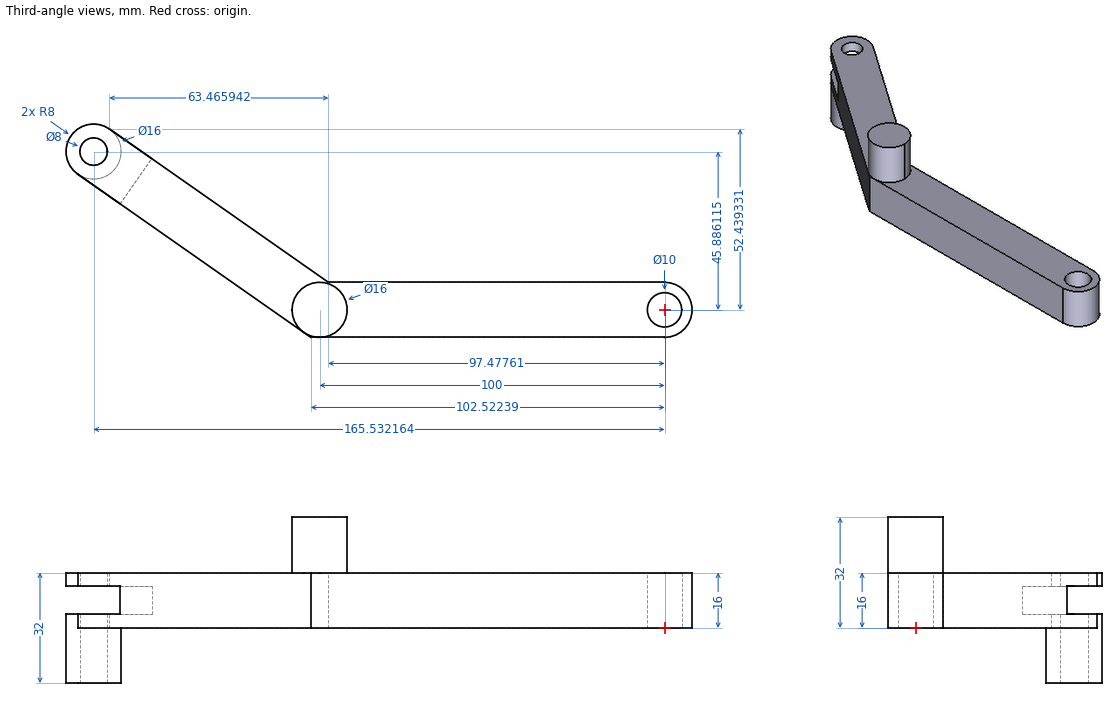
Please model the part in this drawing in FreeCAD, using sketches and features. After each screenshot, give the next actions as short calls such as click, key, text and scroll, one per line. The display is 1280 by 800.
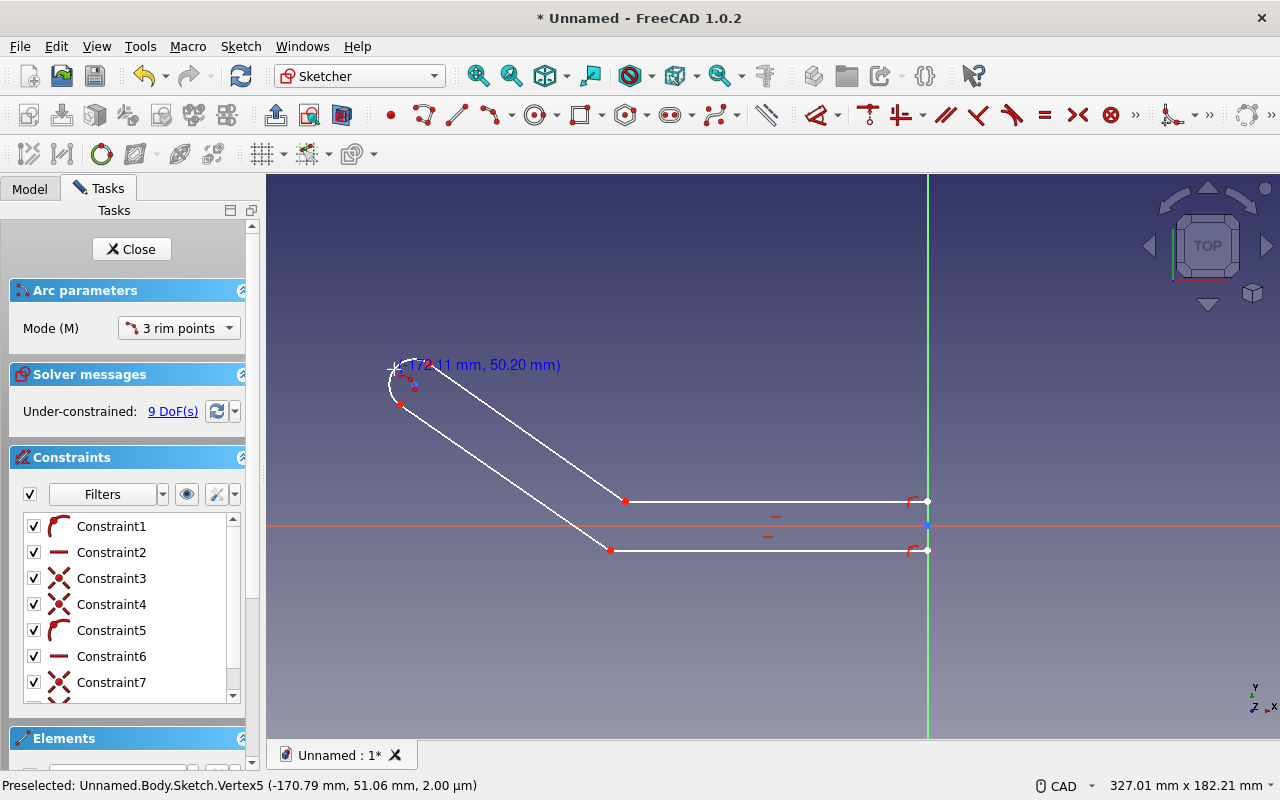
click(928, 551)
click(928, 502)
click(948, 540)
key(Escape)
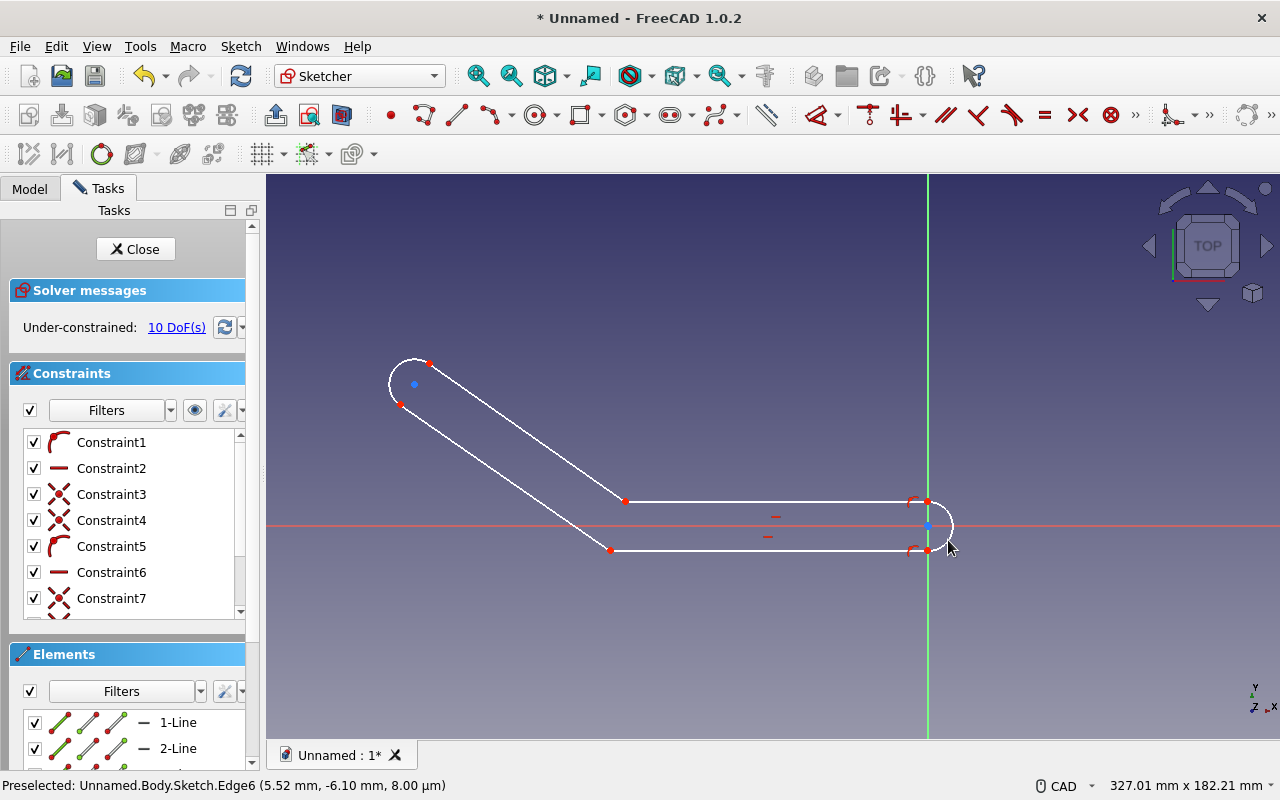
click(837, 502)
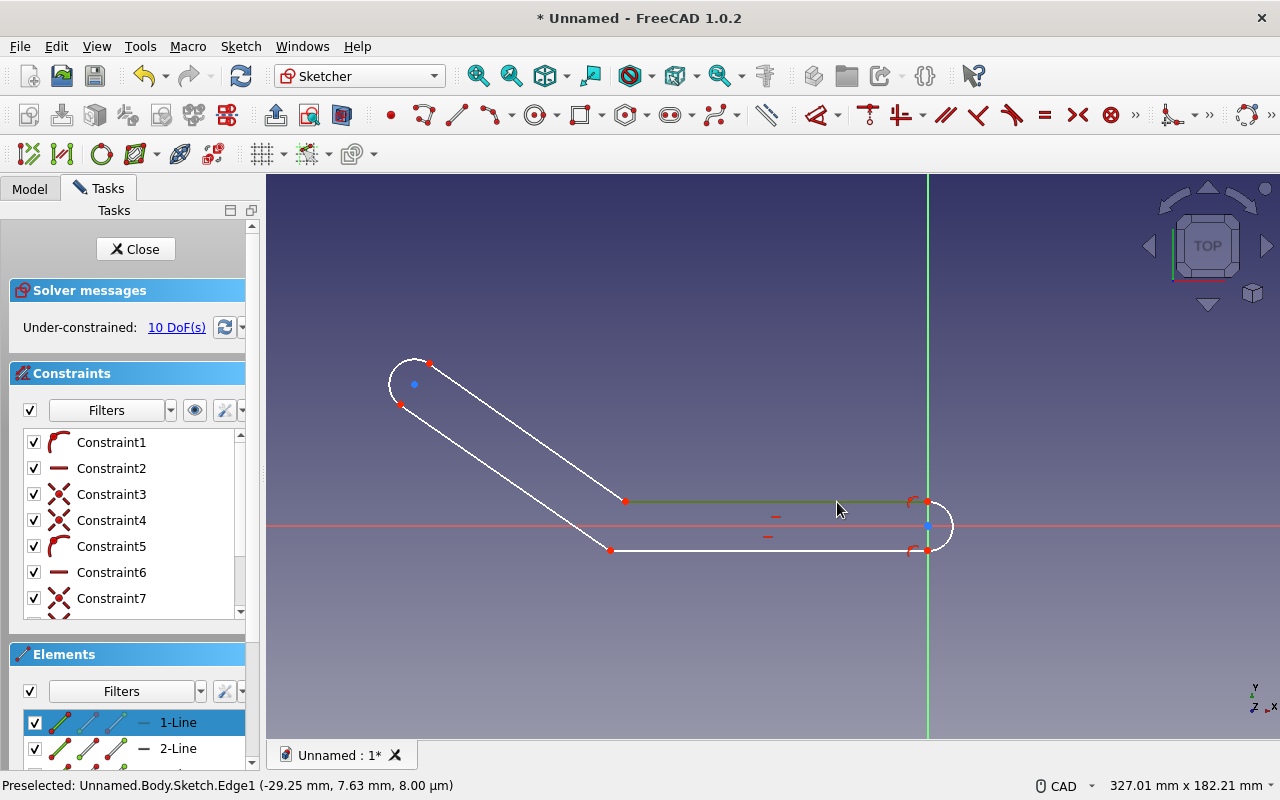
click(948, 541)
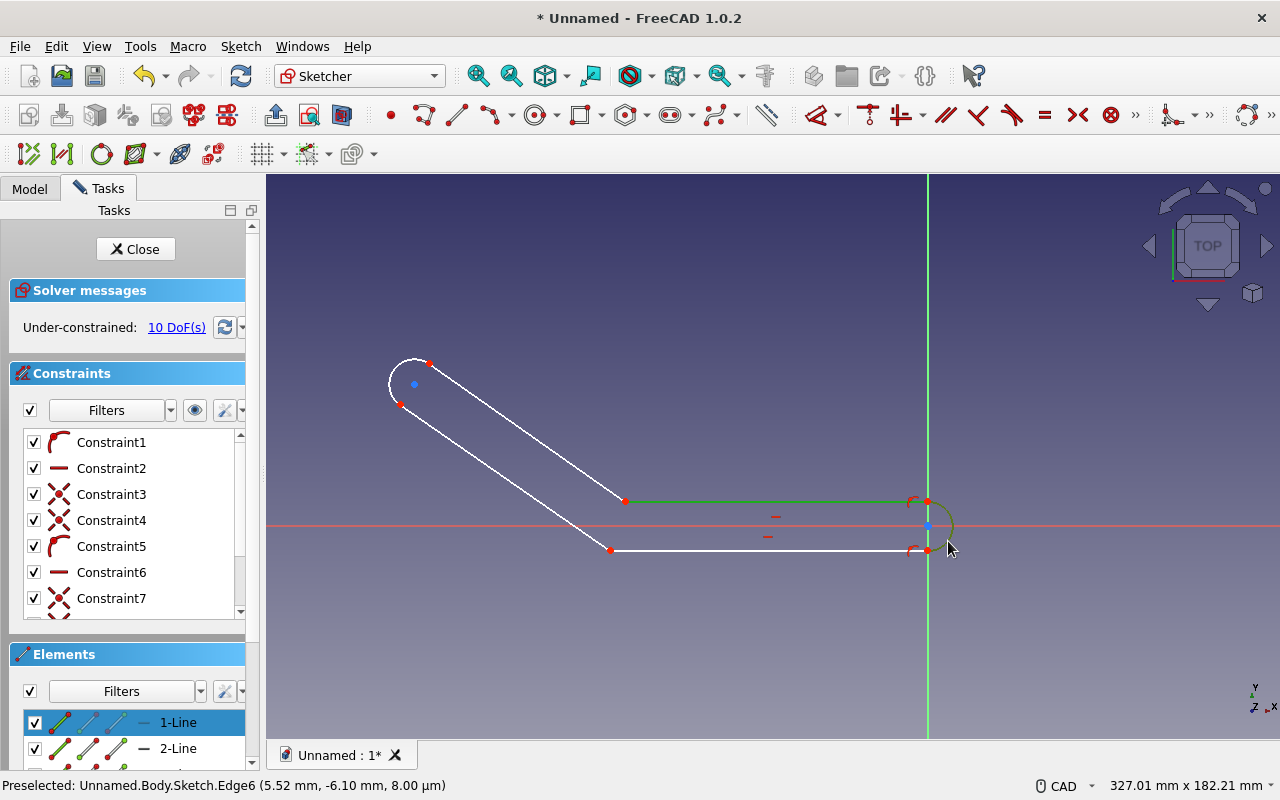
click(1012, 116)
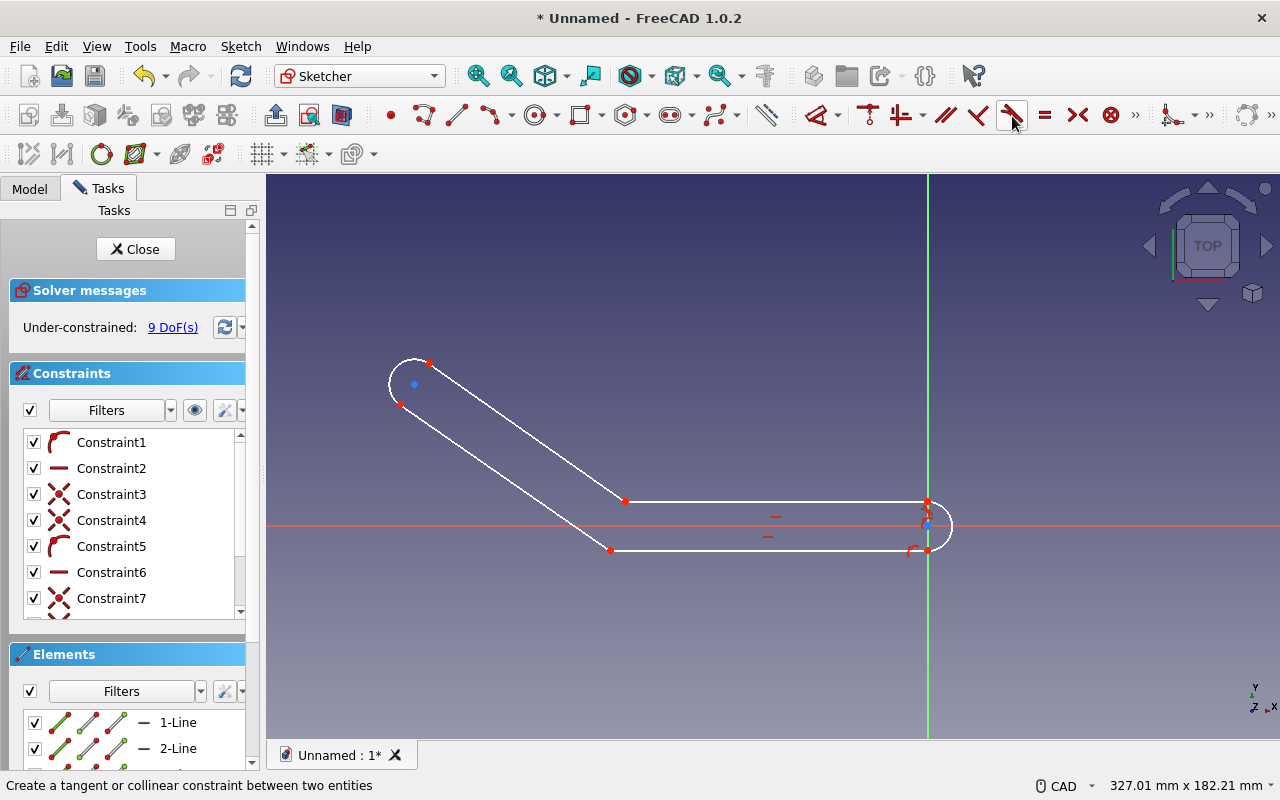
click(566, 461)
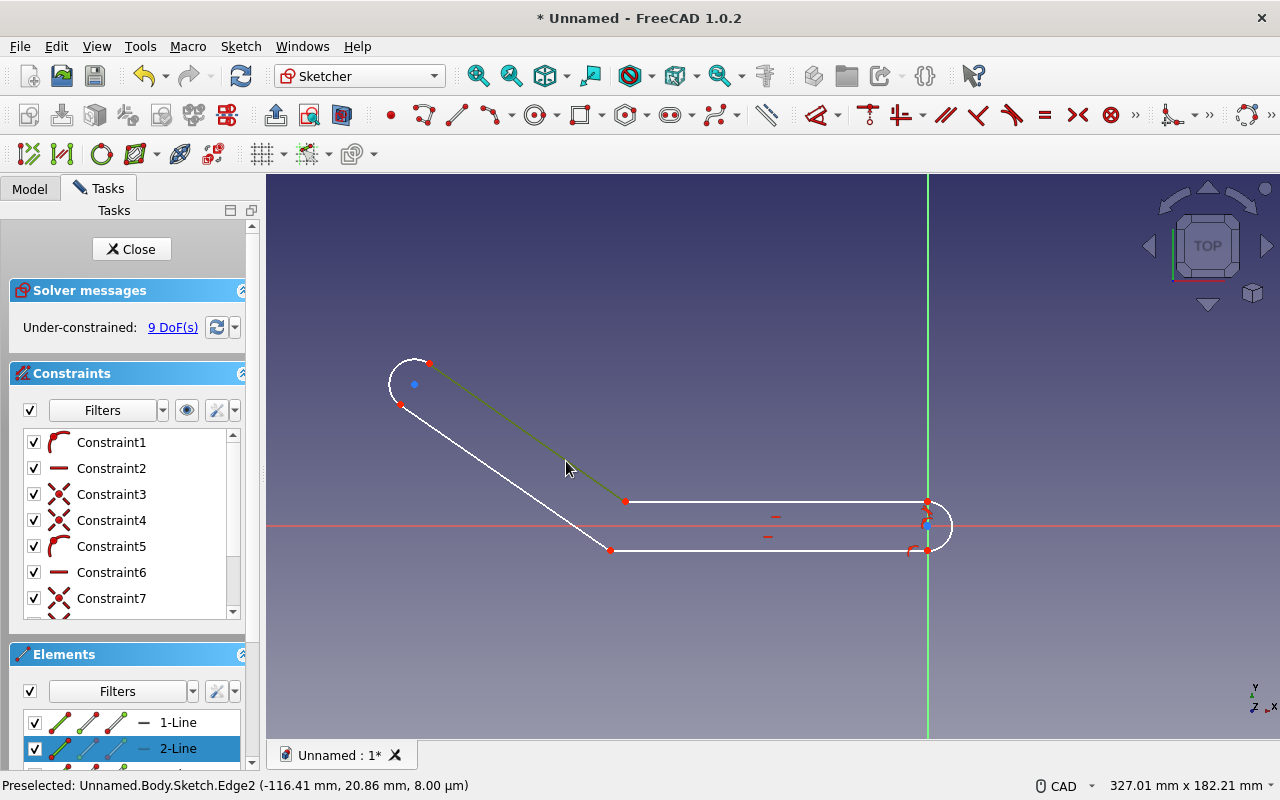
click(406, 361)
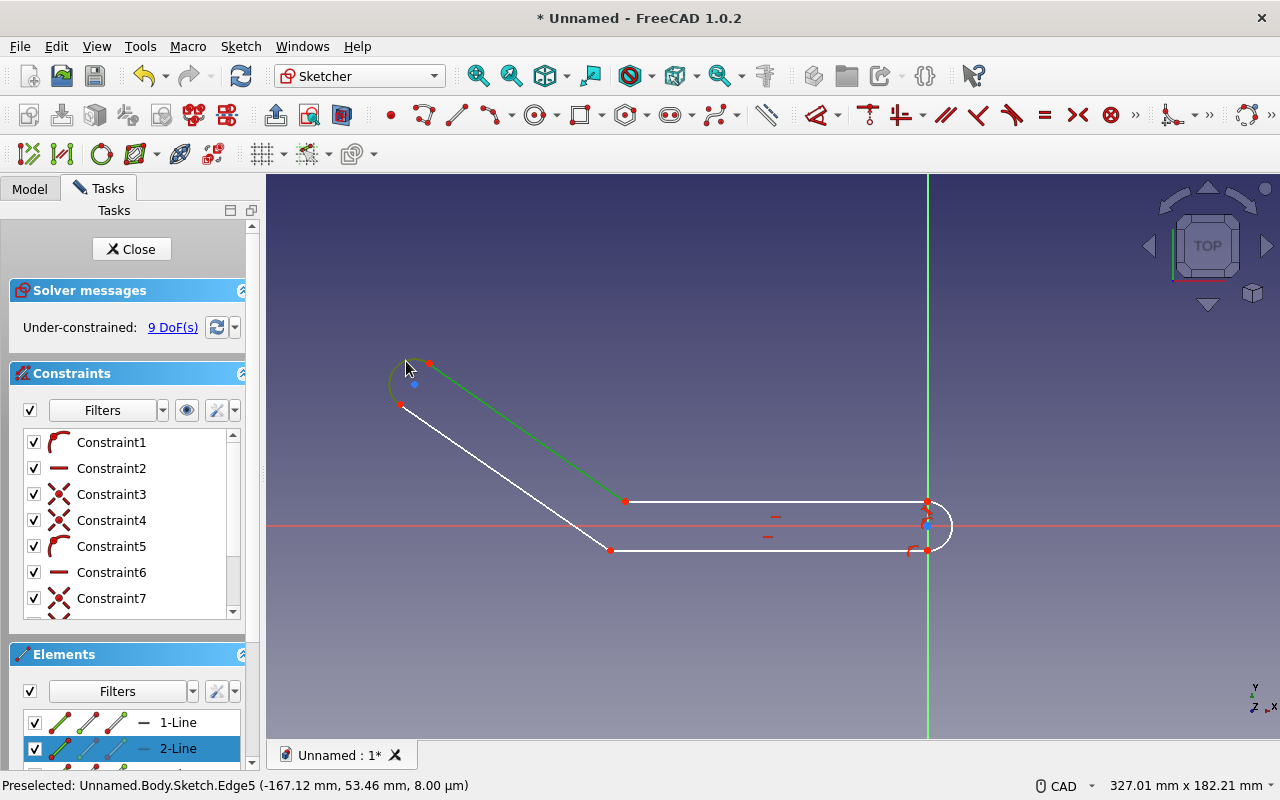
click(1012, 116)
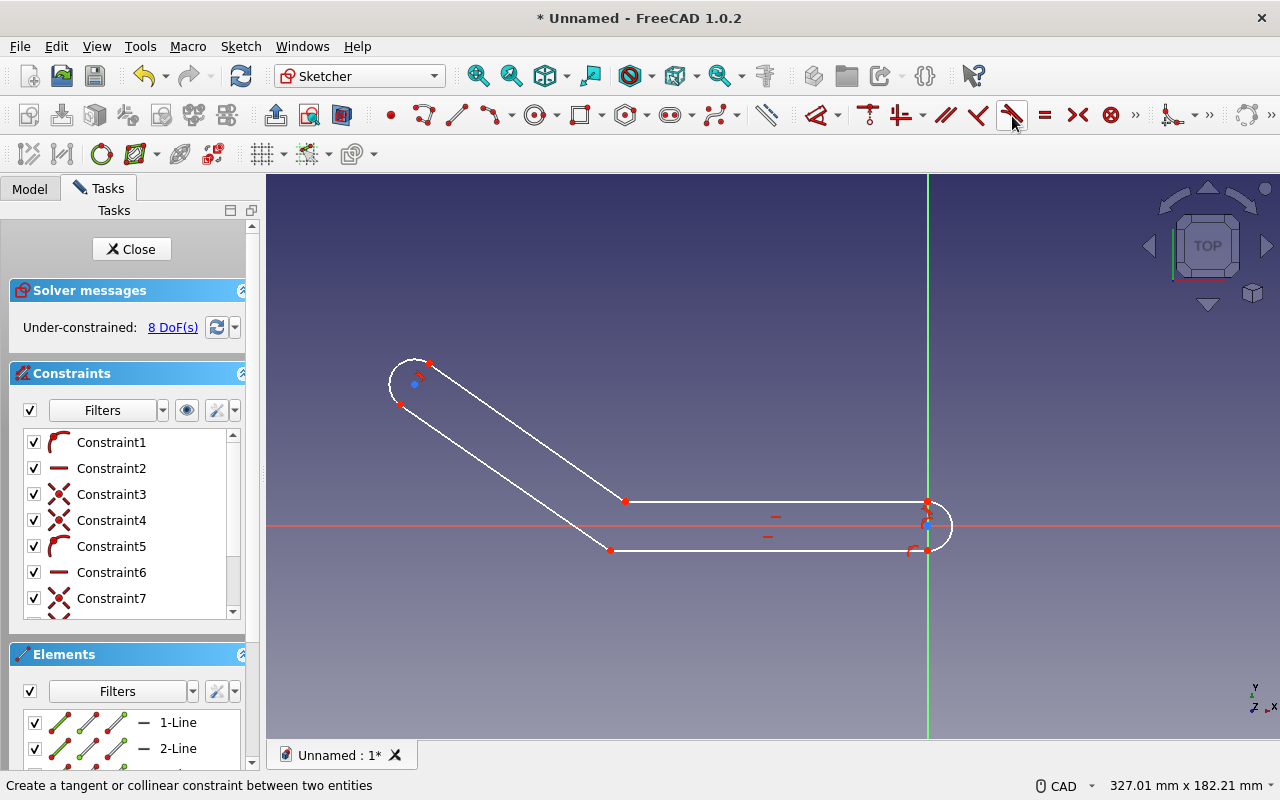
click(463, 449)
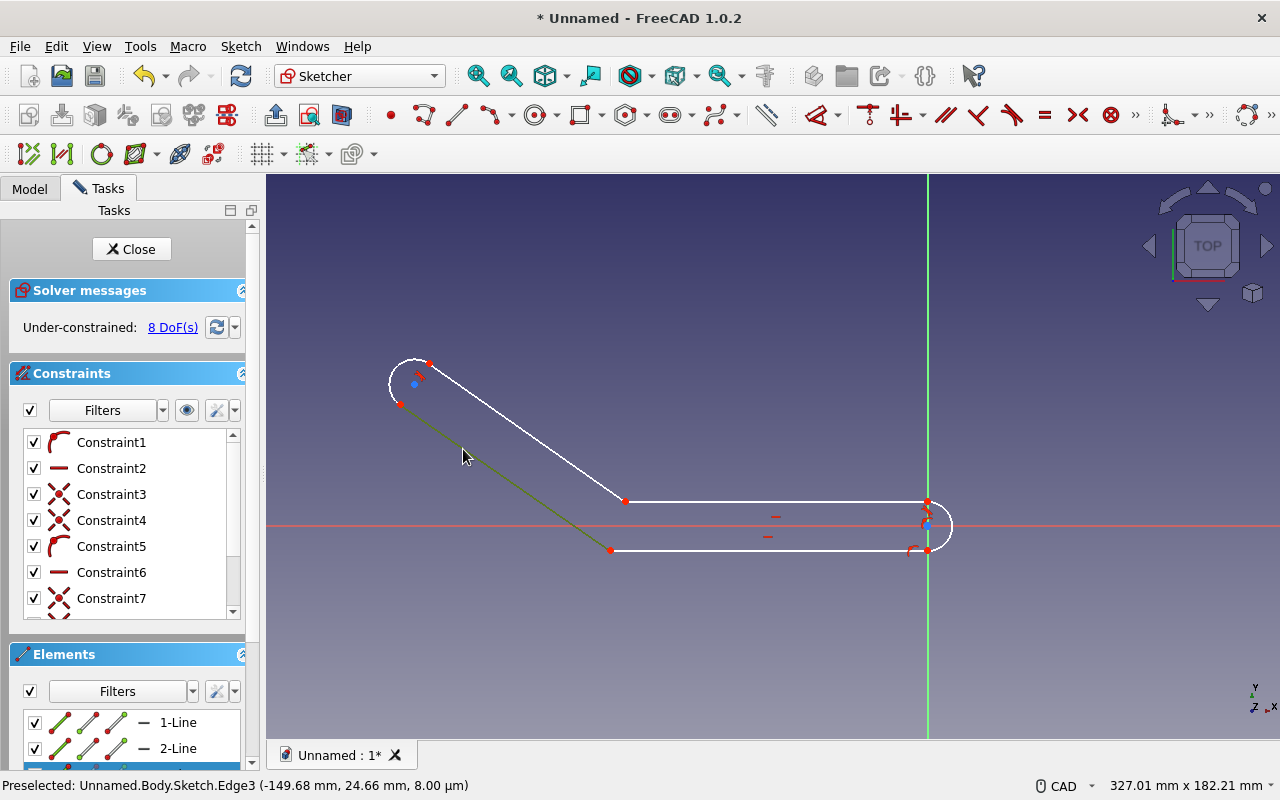
click(406, 361)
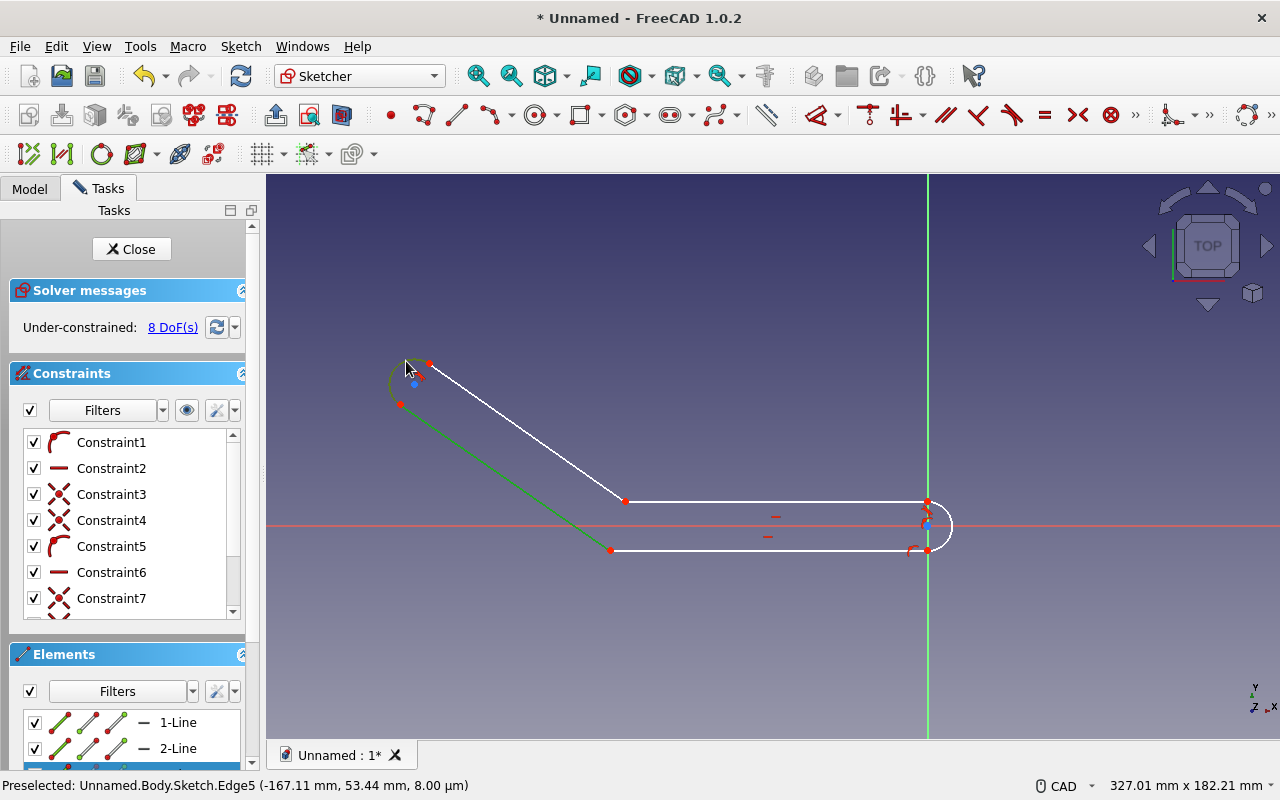
click(1012, 116)